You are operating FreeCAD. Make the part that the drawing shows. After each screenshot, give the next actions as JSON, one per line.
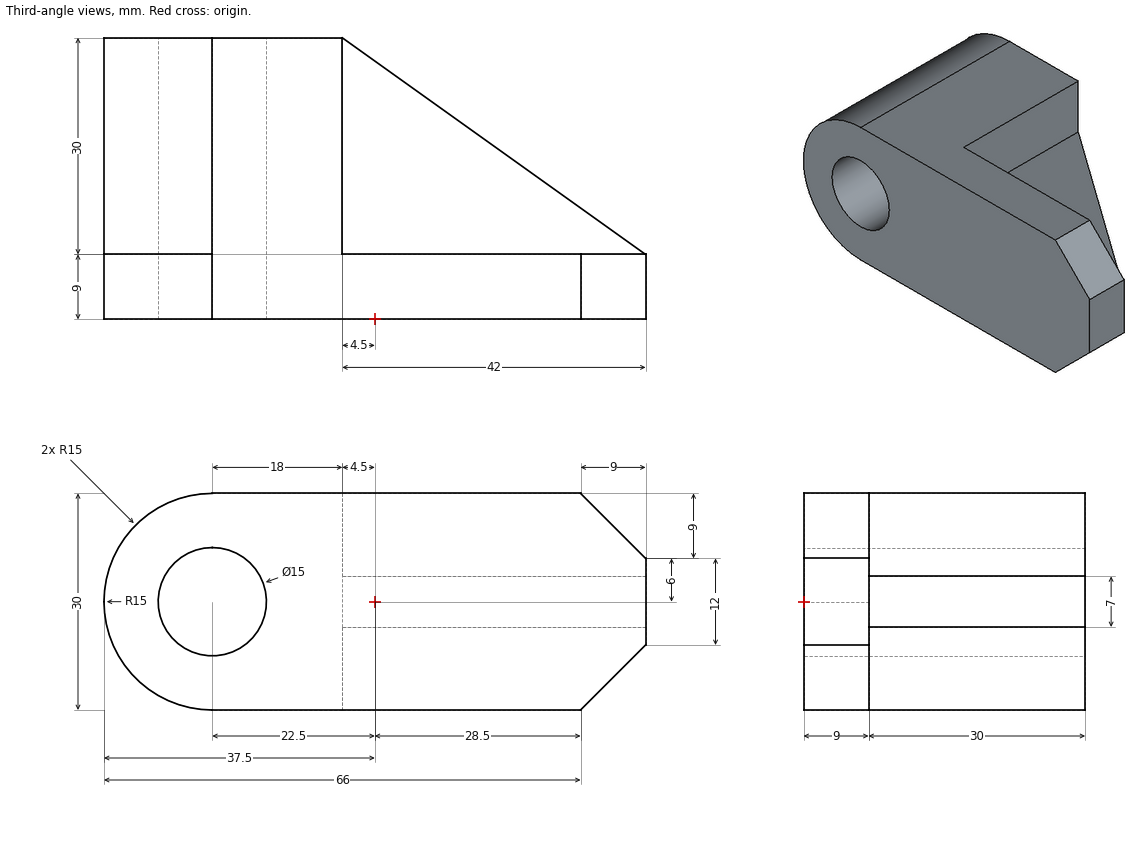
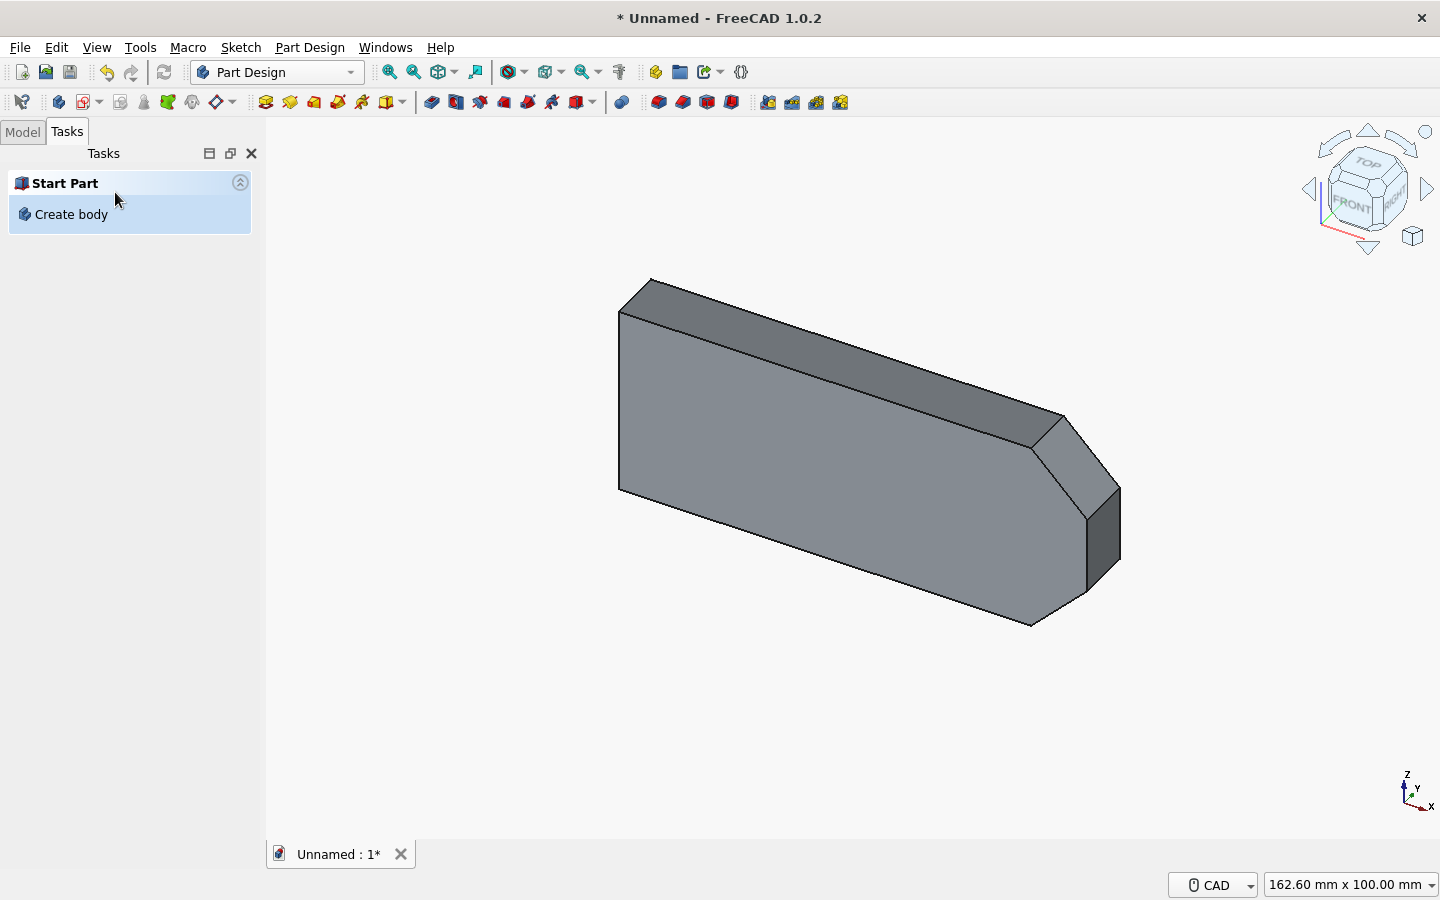
{"action": "key", "text": "4"}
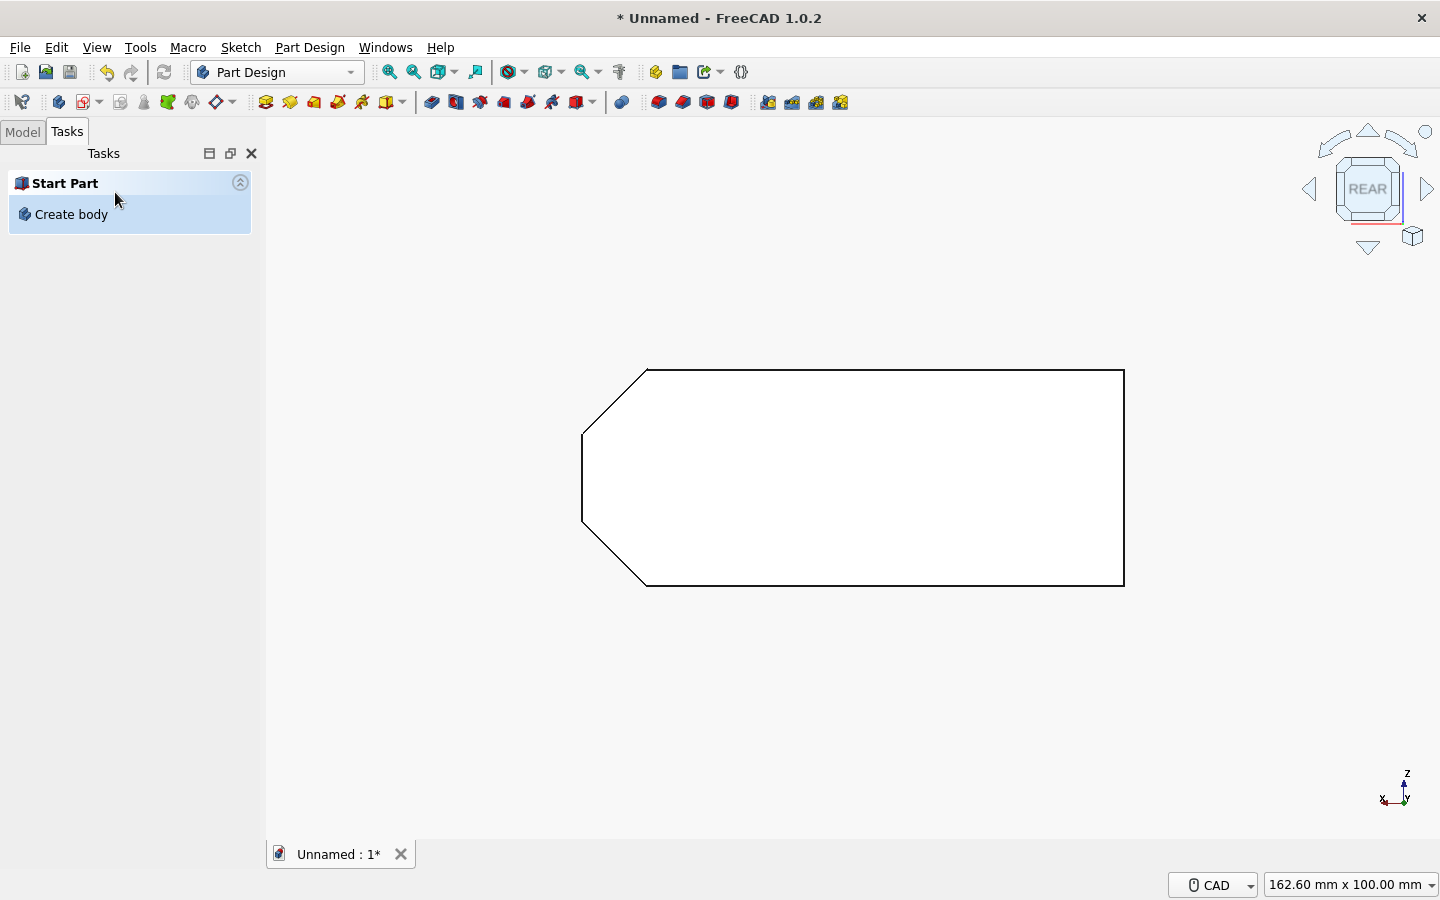
{"action": "left_click", "coordinate": [698, 477]}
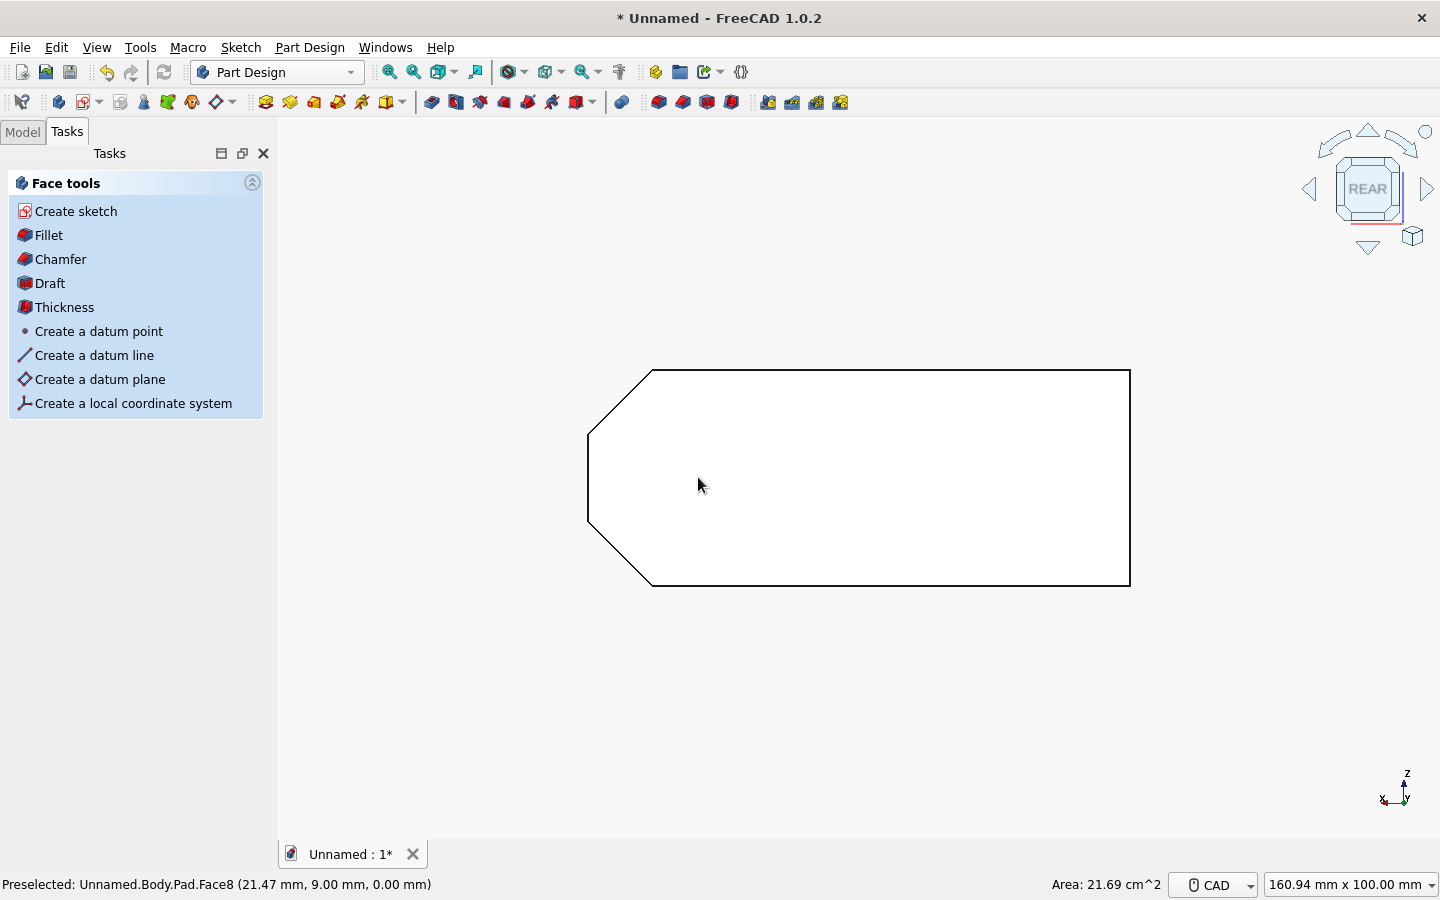
{"action": "left_click", "coordinate": [84, 102]}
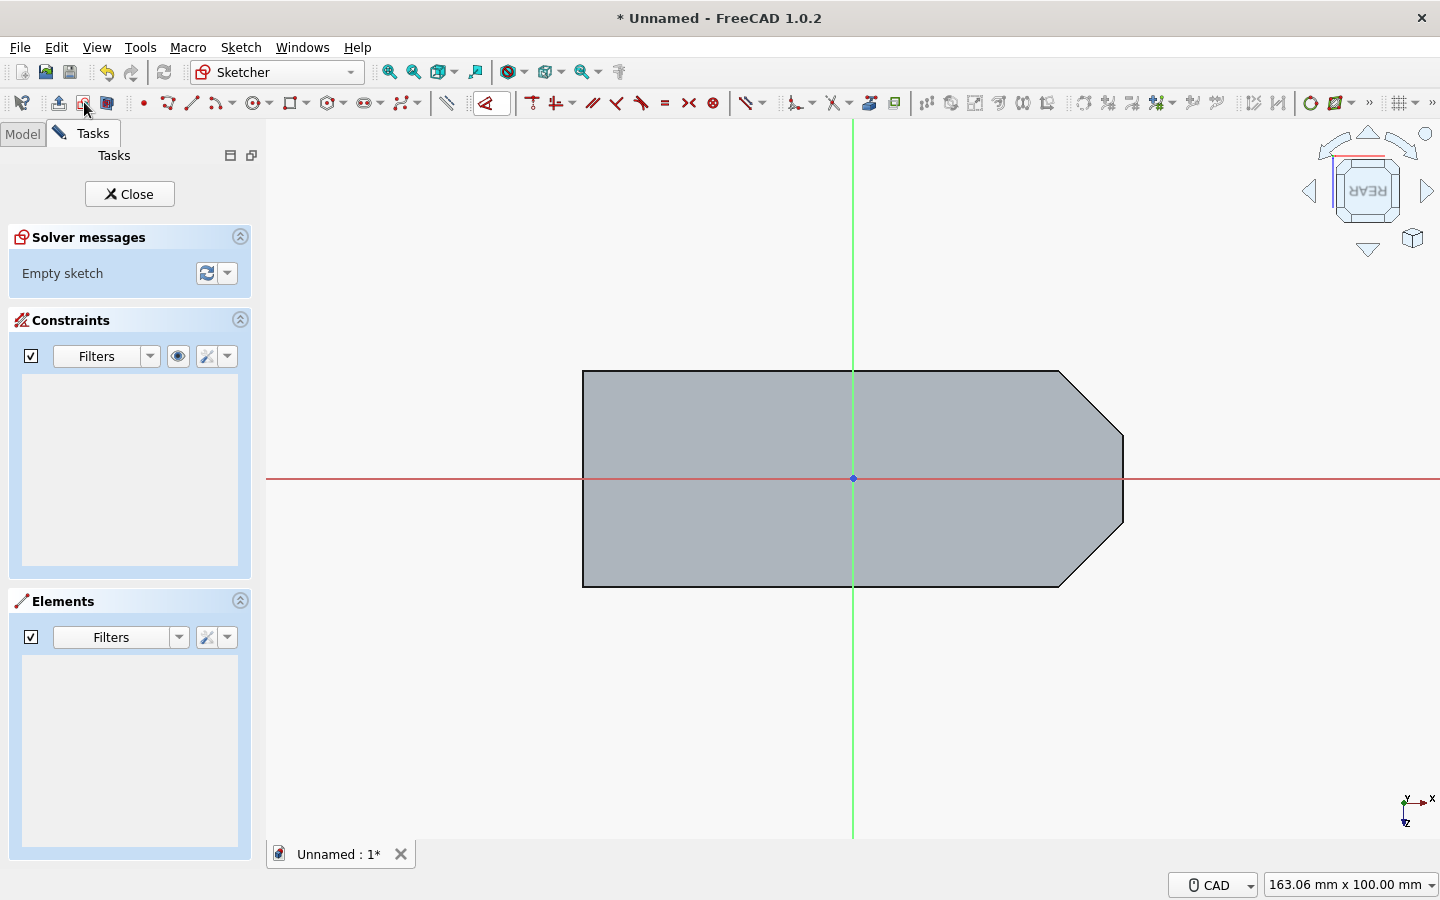
{"action": "scroll", "coordinate": [664, 479], "scroll_direction": "up", "scroll_amount": 4}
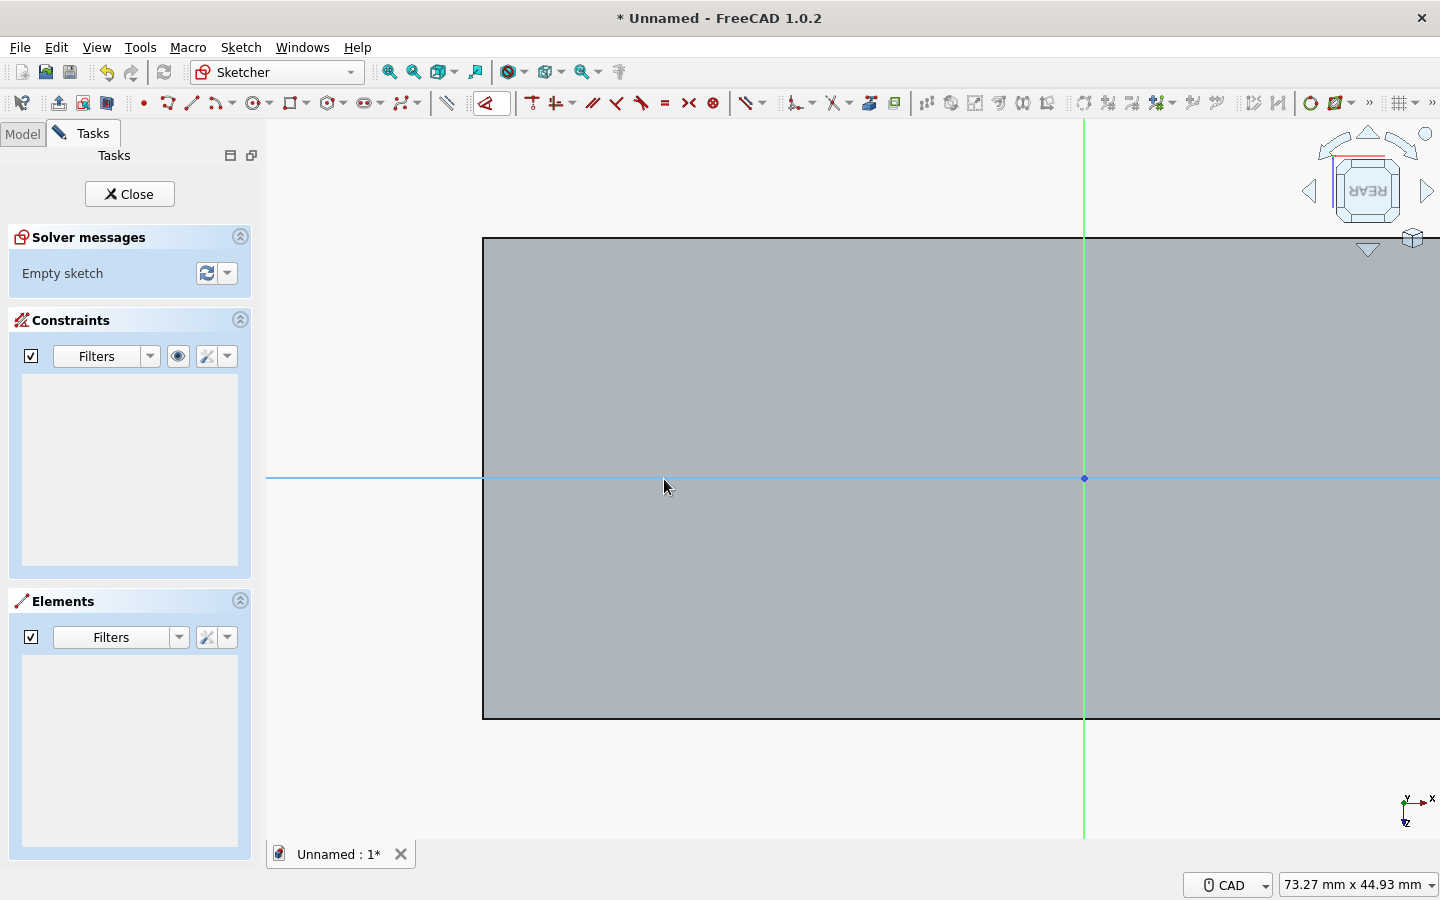
{"action": "key", "text": "g m"}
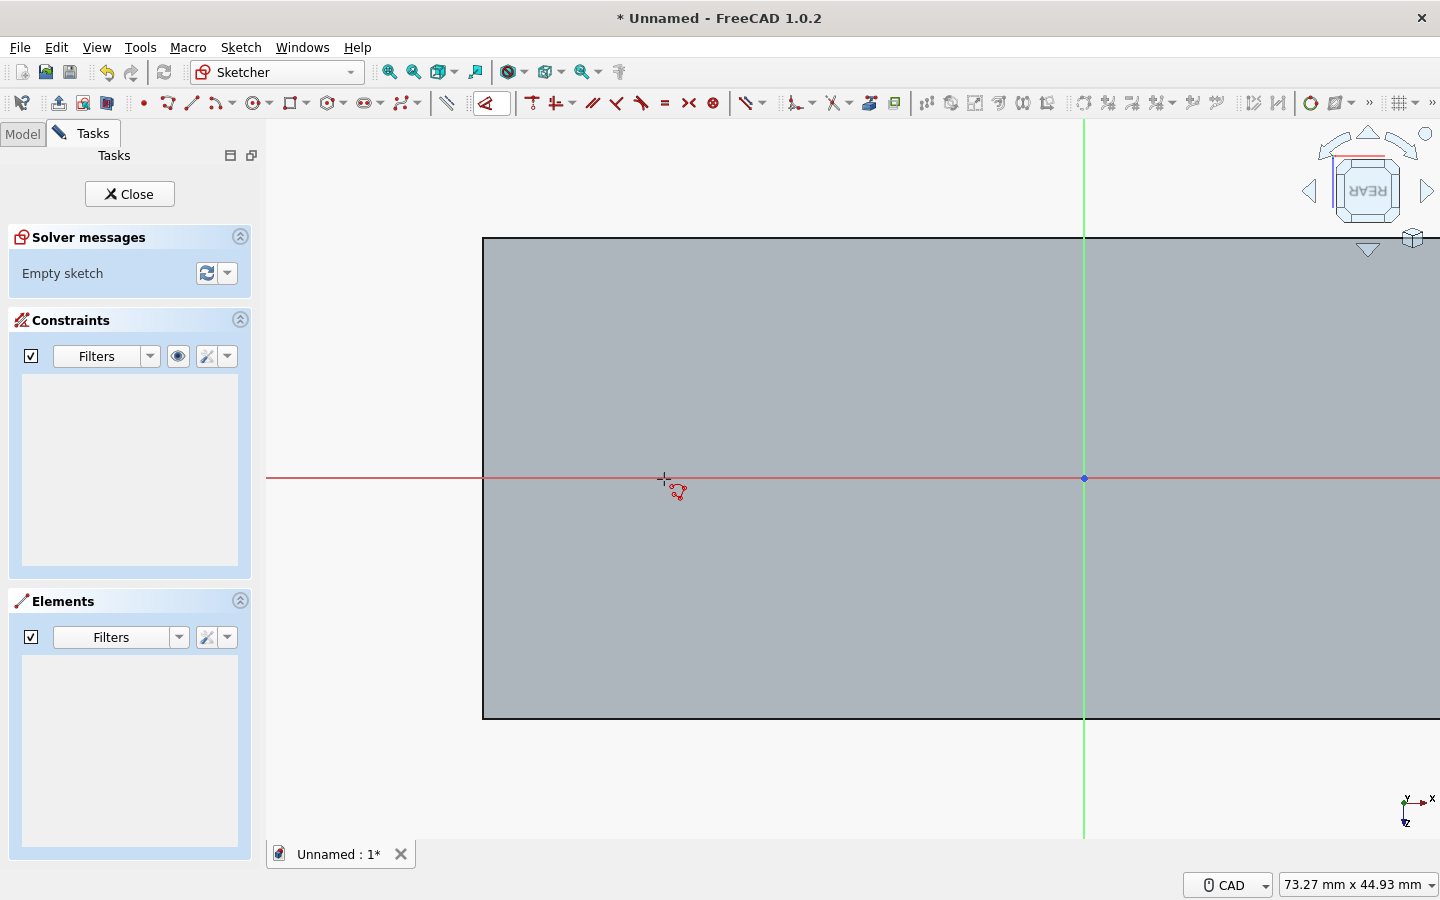
{"action": "left_click", "coordinate": [483, 478]}
{"action": "left_click", "coordinate": [483, 719]}
{"action": "left_click", "coordinate": [724, 719]}
{"action": "right_click", "coordinate": [724, 719]}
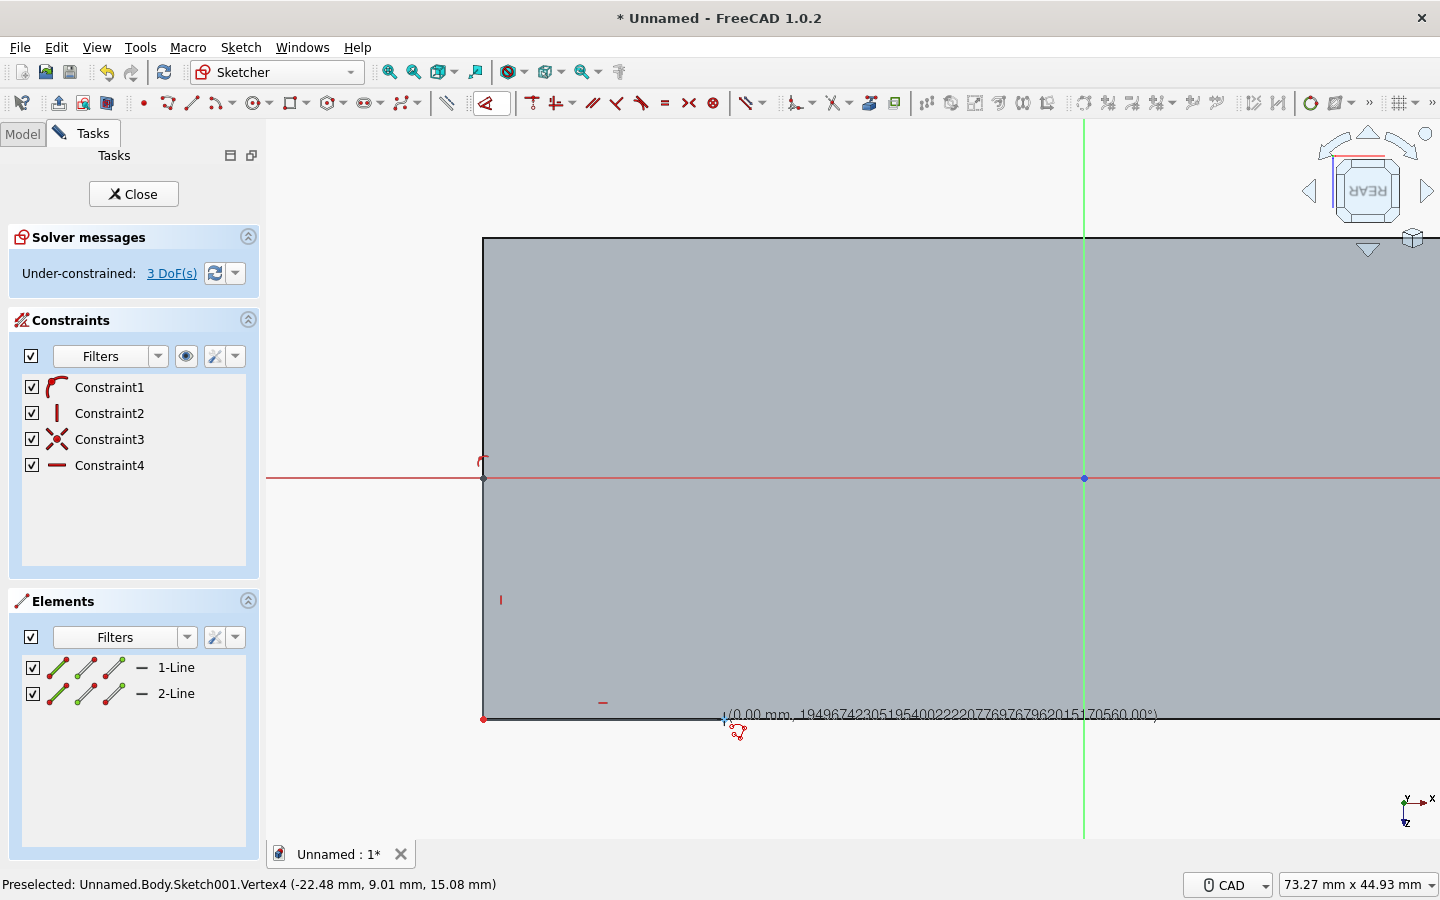
{"action": "left_click", "coordinate": [234, 104]}